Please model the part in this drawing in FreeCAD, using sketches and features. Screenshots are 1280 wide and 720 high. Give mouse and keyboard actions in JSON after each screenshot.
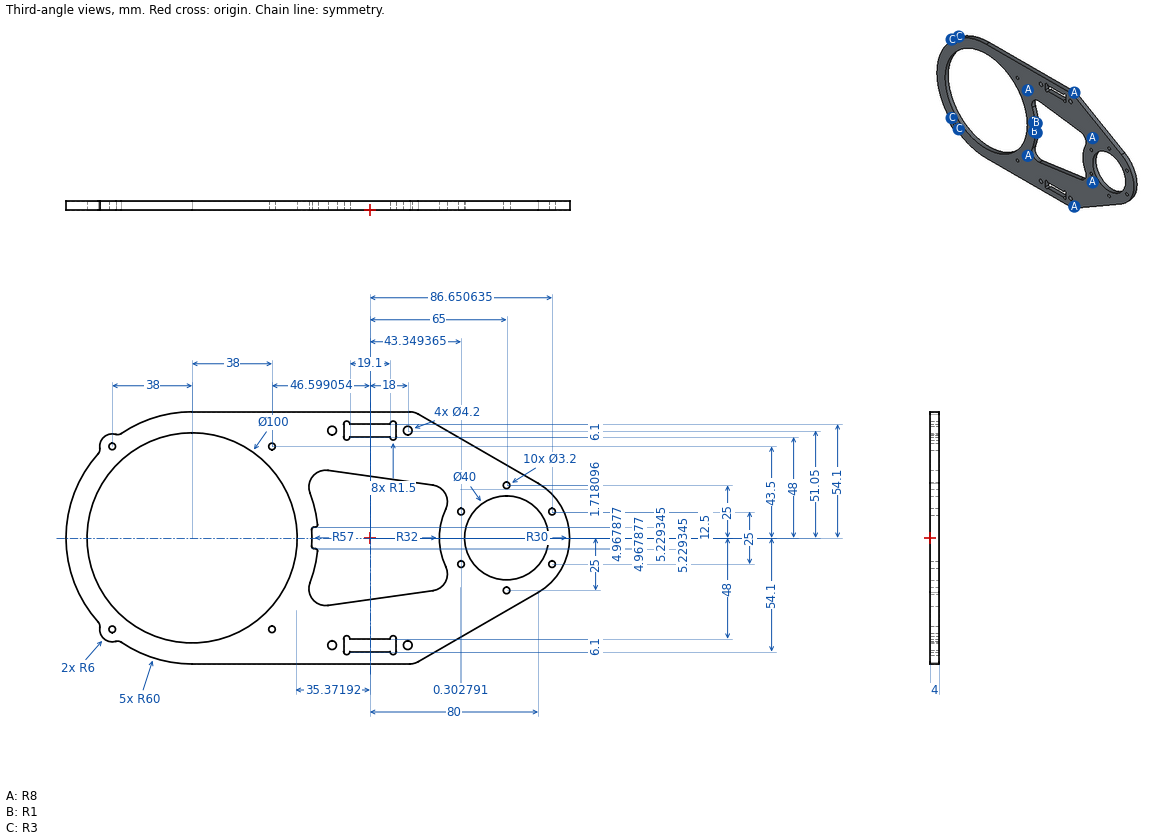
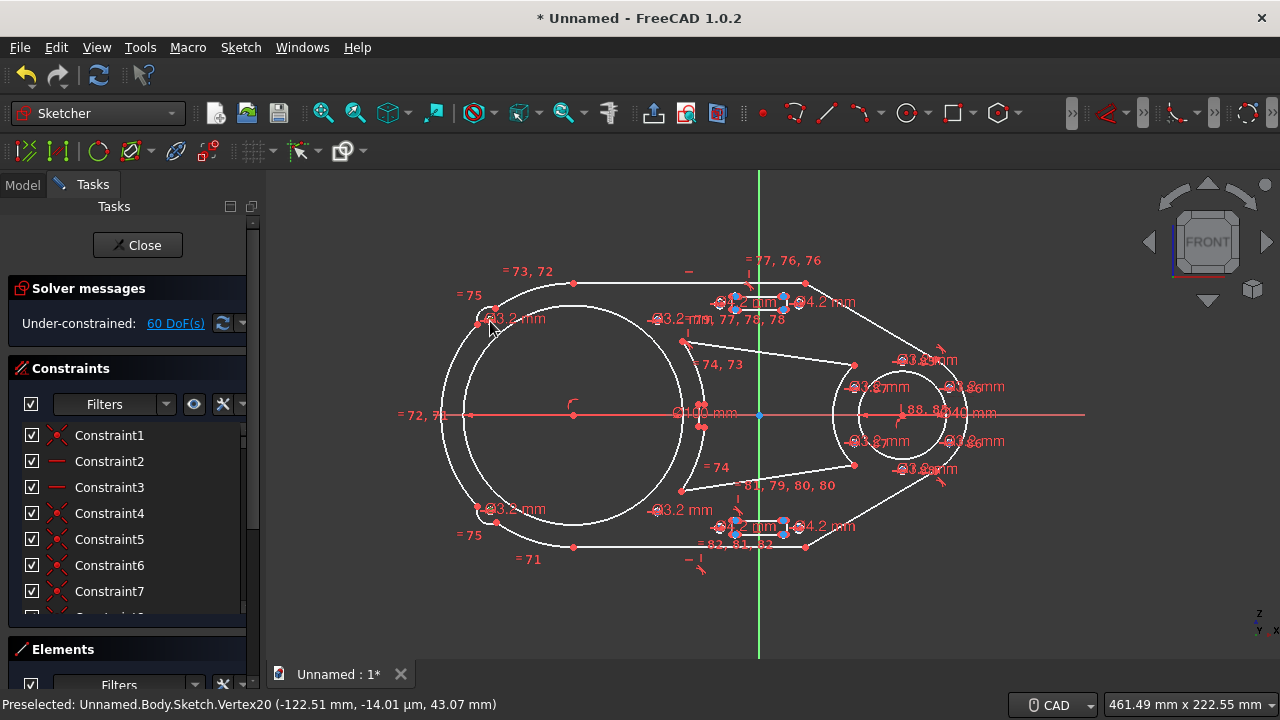
{"action": "left_click", "coordinate": [529, 415]}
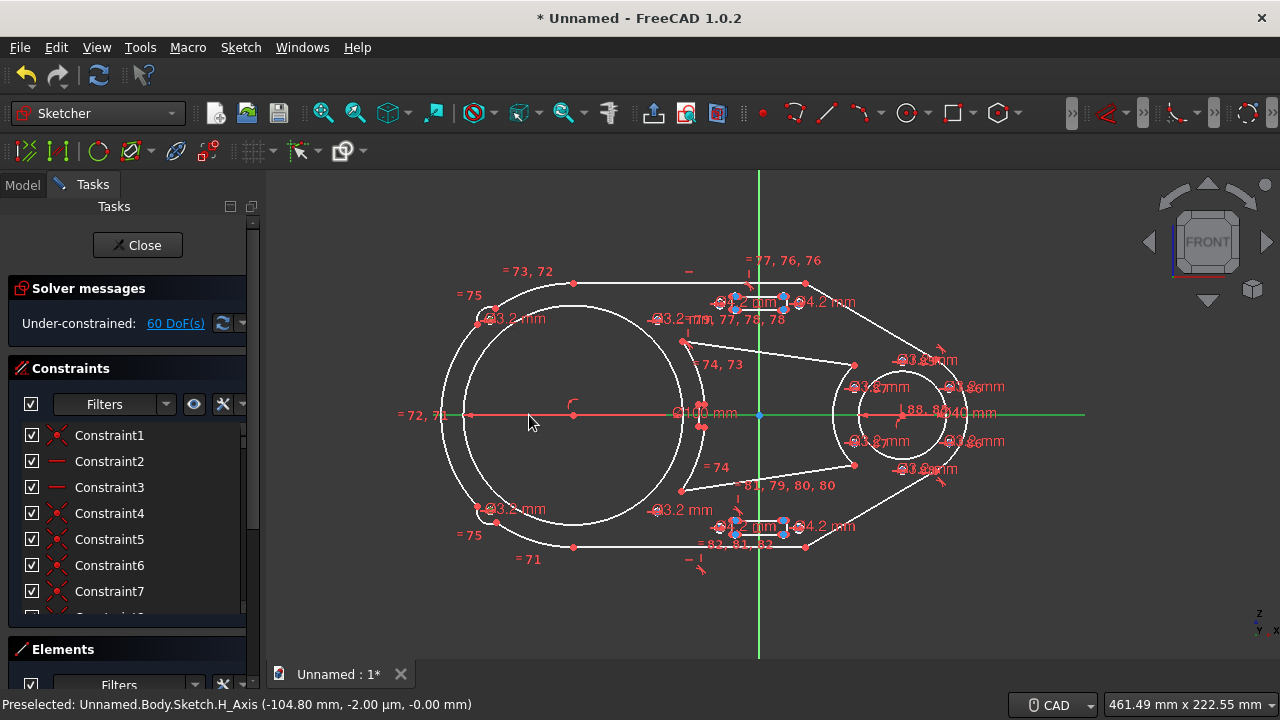
{"action": "key", "text": "s"}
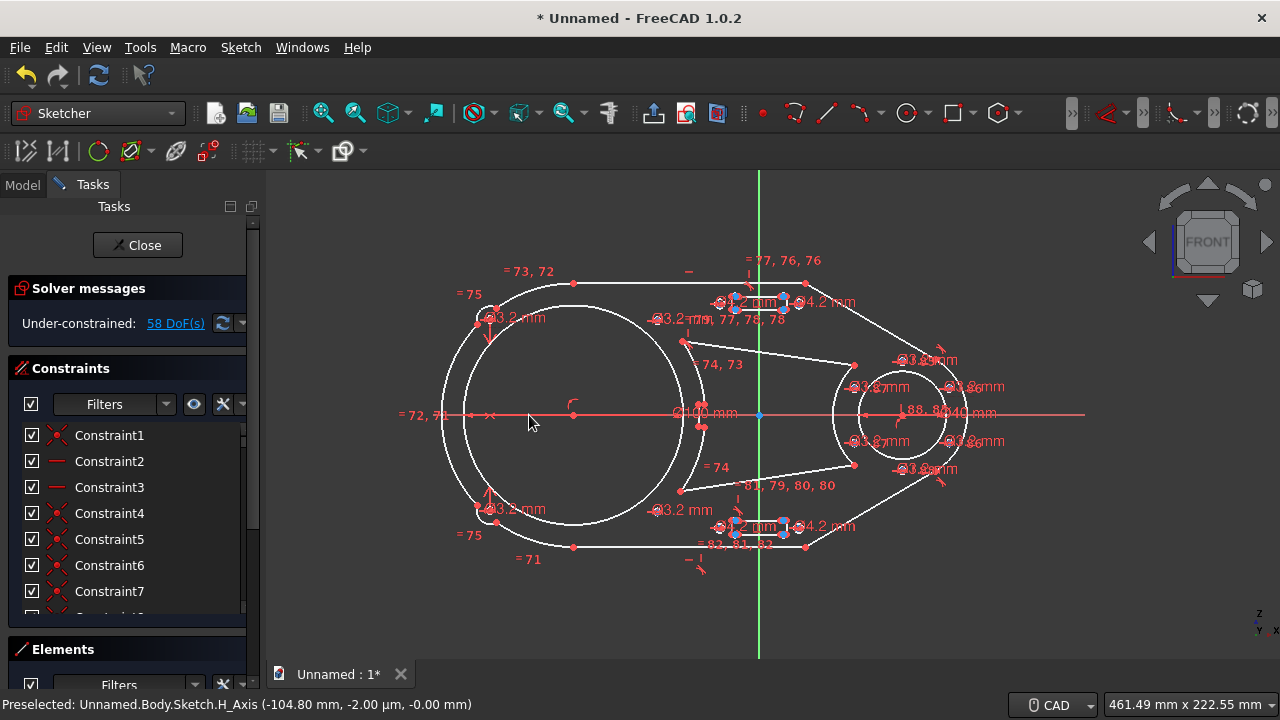
{"action": "scroll", "coordinate": [784, 297], "scroll_direction": "up", "scroll_amount": 7}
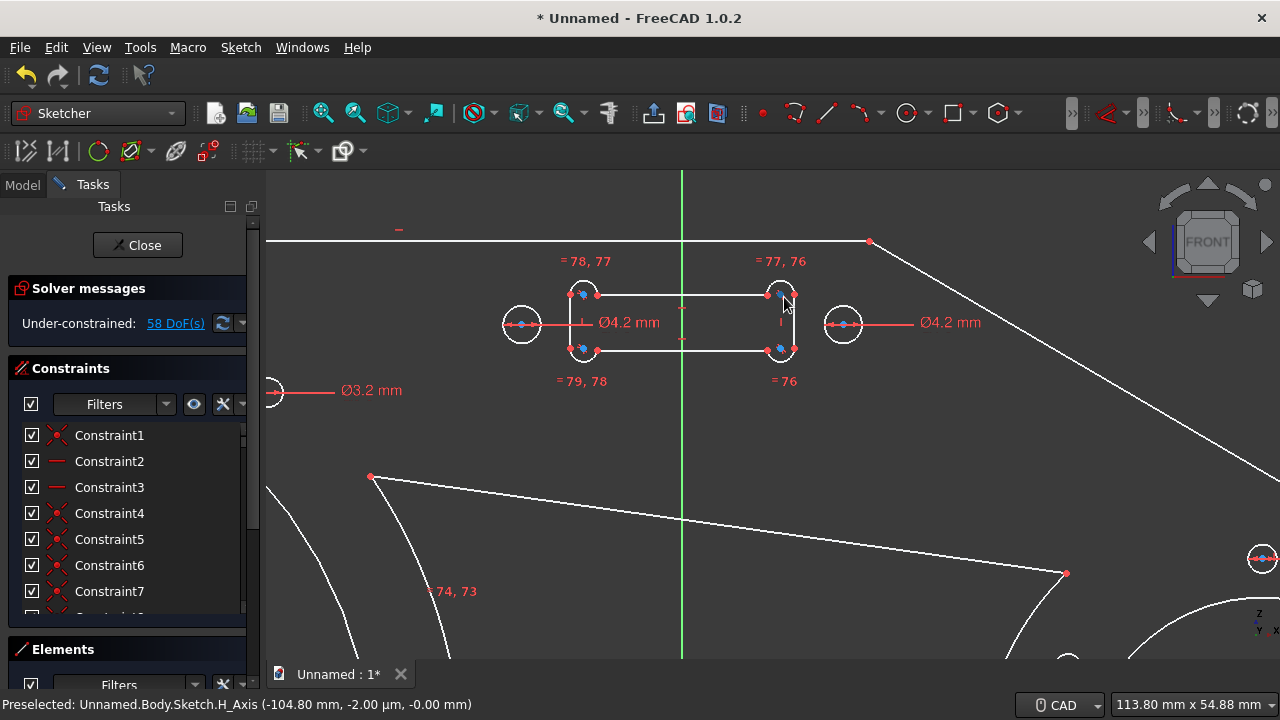
{"action": "left_click", "coordinate": [781, 294]}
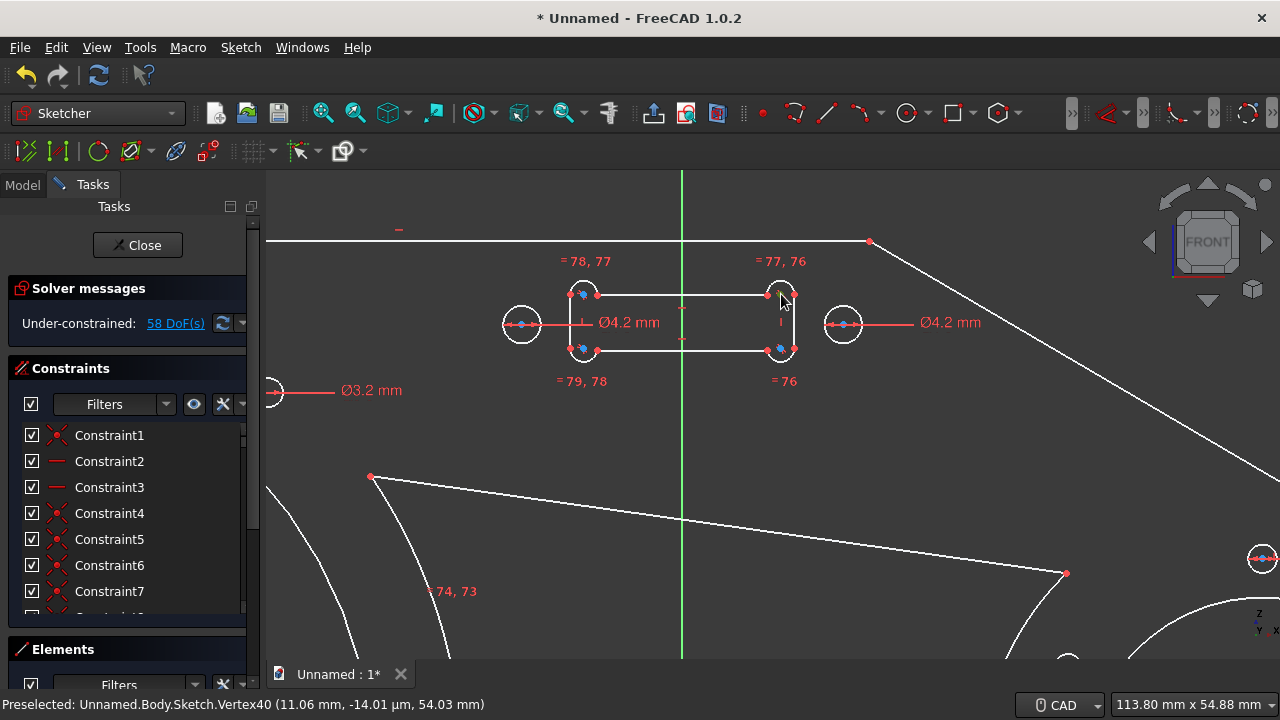
{"action": "left_click", "coordinate": [584, 294]}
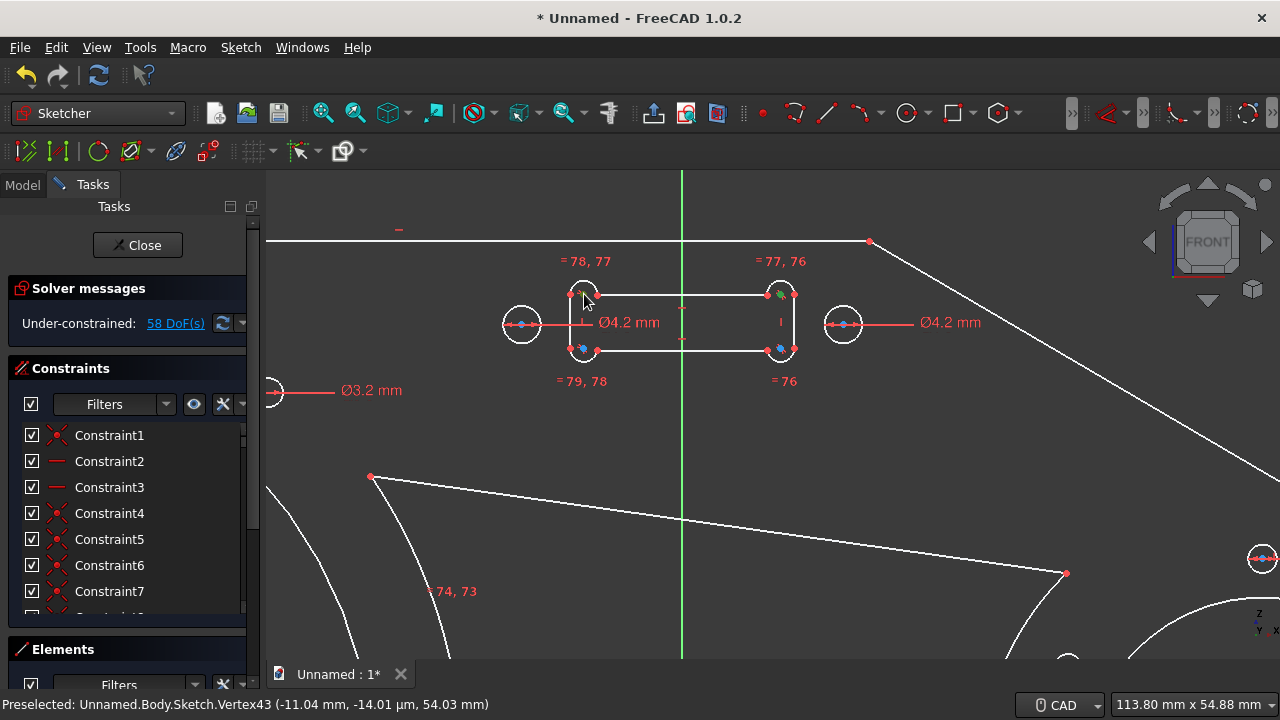
{"action": "left_click", "coordinate": [682, 600]}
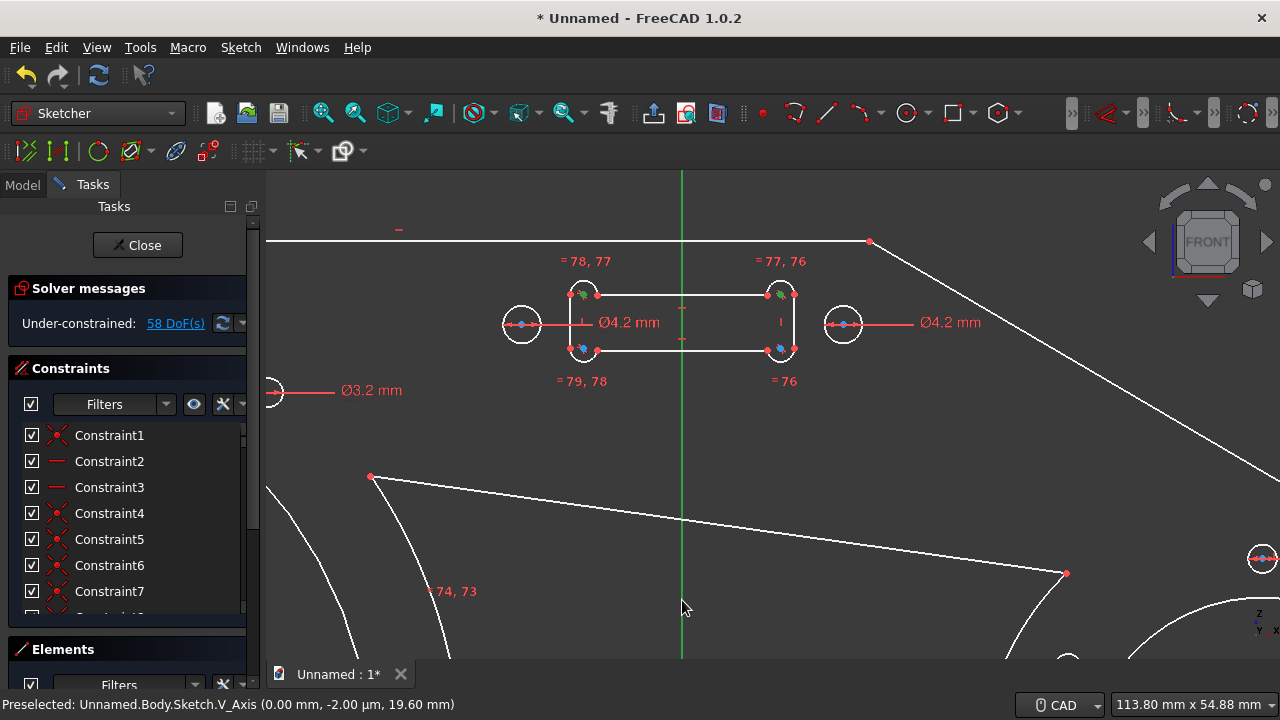
{"action": "key", "text": "s"}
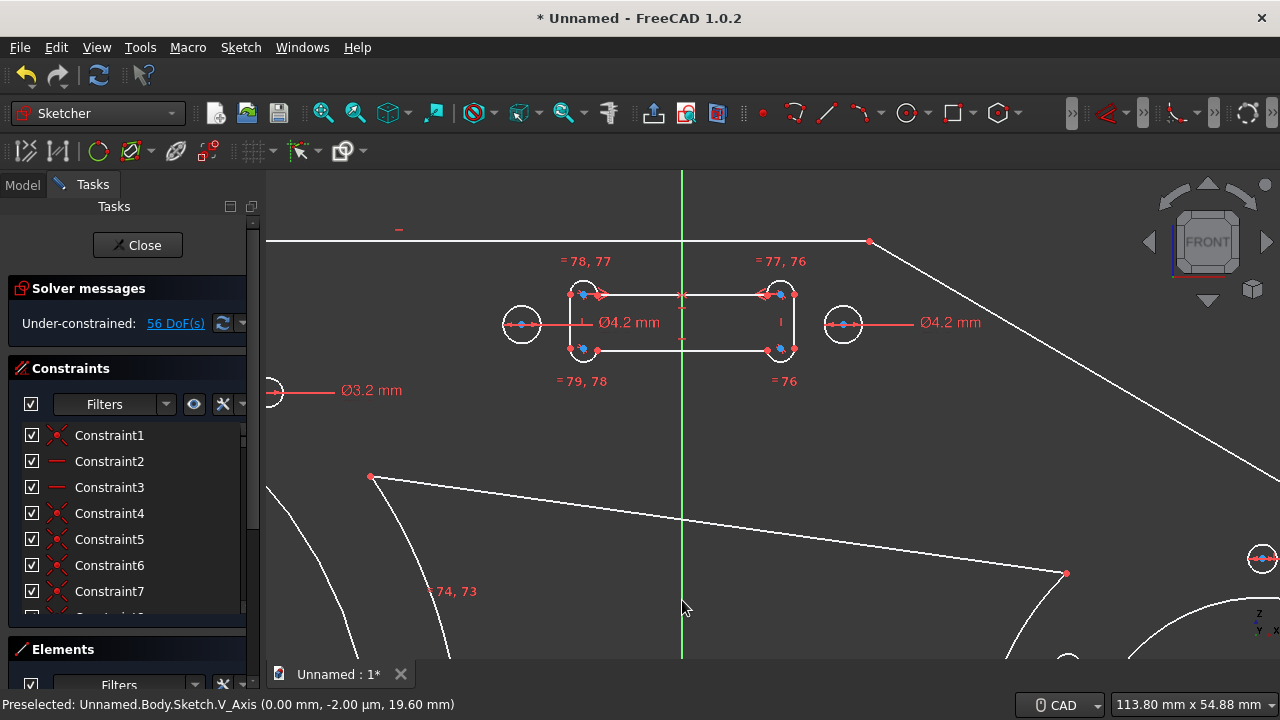
{"action": "left_click", "coordinate": [781, 294]}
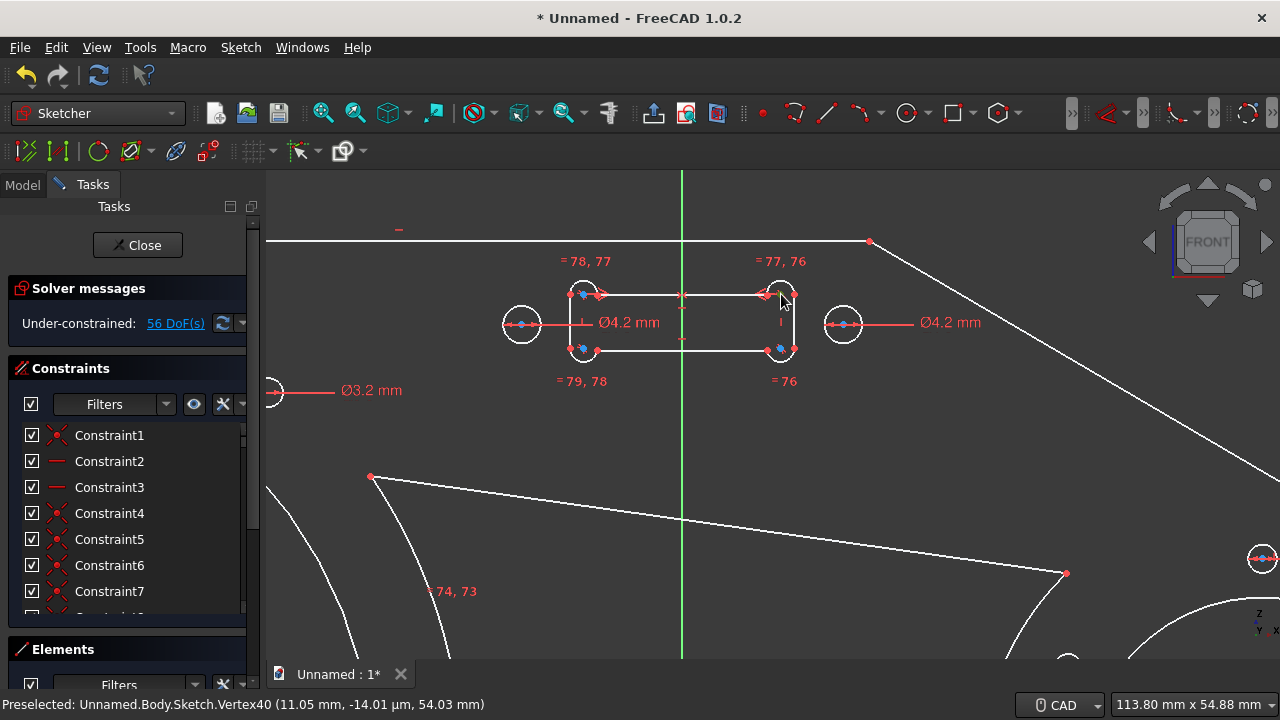
{"action": "scroll", "coordinate": [784, 296], "scroll_direction": "down", "scroll_amount": 7}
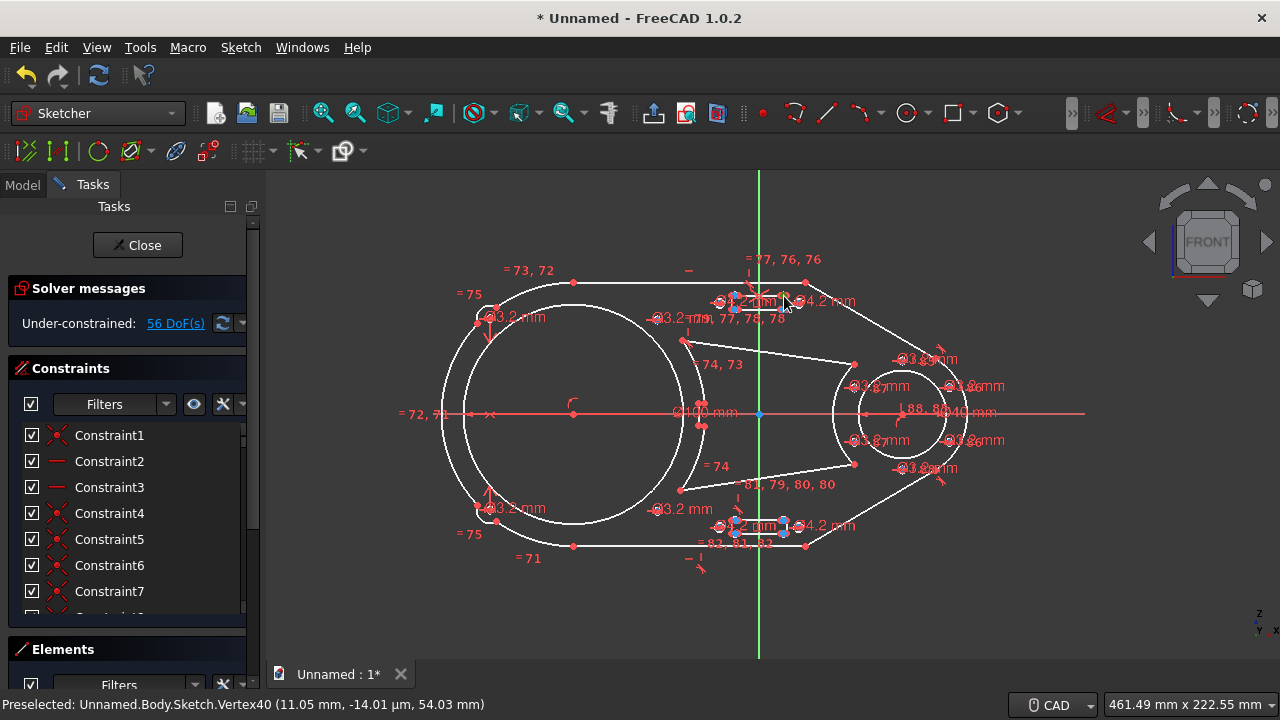
{"action": "scroll", "coordinate": [784, 534], "scroll_direction": "up", "scroll_amount": 7}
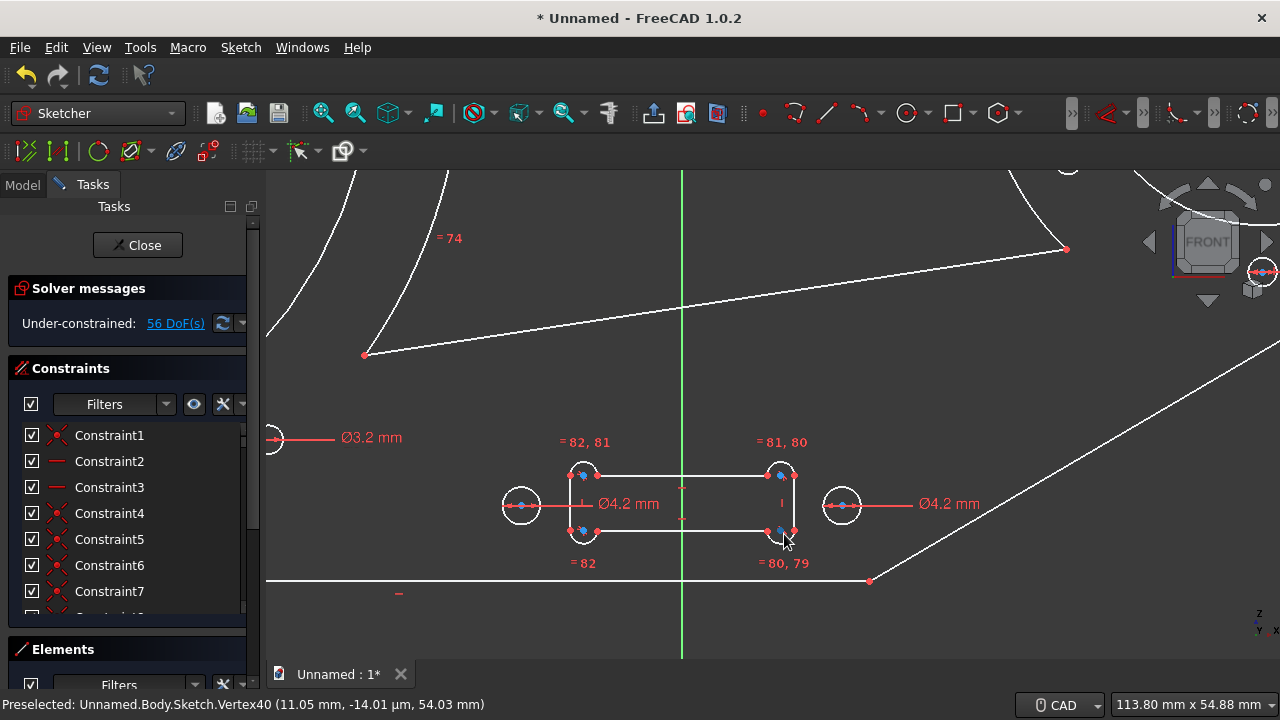
{"action": "left_click", "coordinate": [781, 530]}